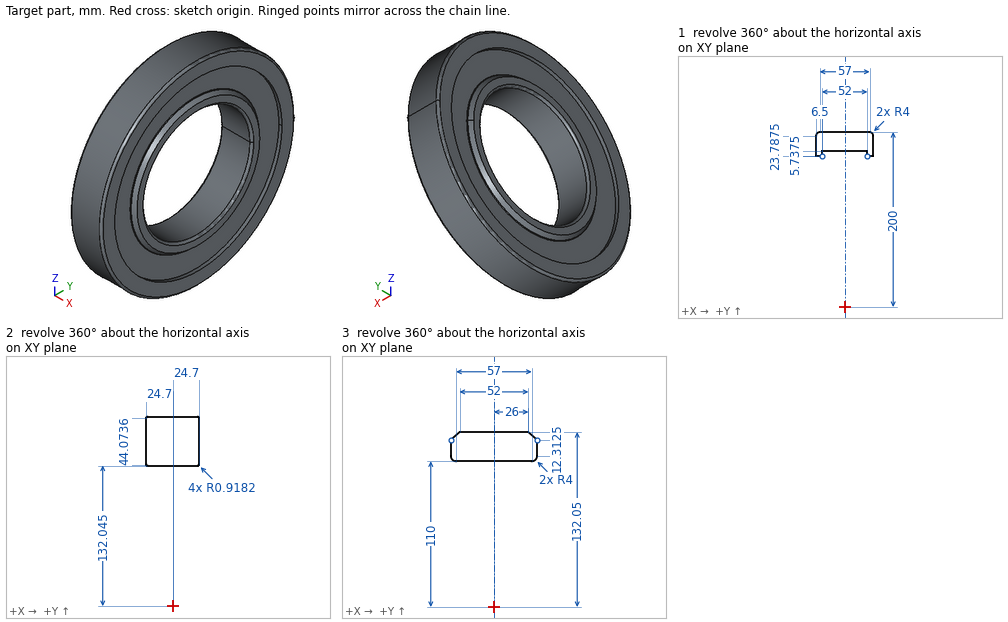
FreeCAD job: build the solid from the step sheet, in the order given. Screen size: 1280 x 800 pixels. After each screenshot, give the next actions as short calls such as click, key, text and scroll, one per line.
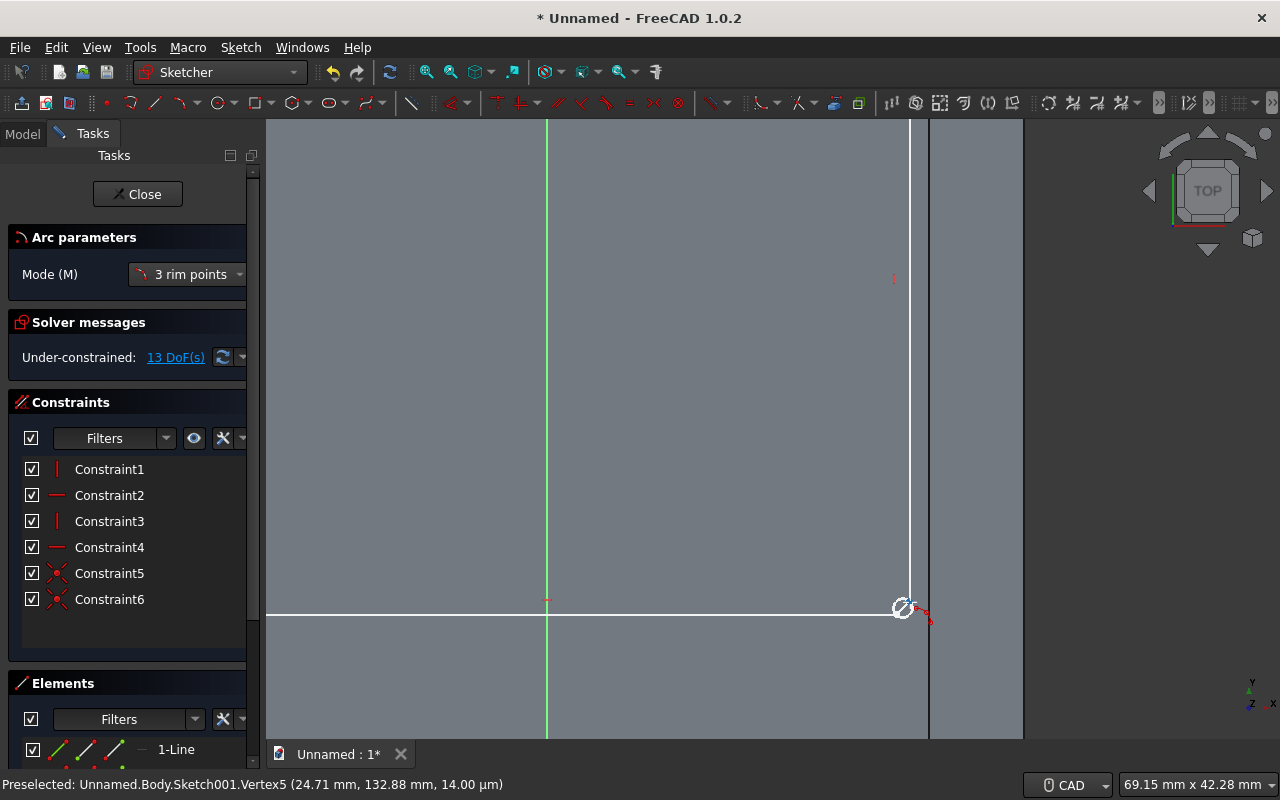
scroll(906, 610, up, 7)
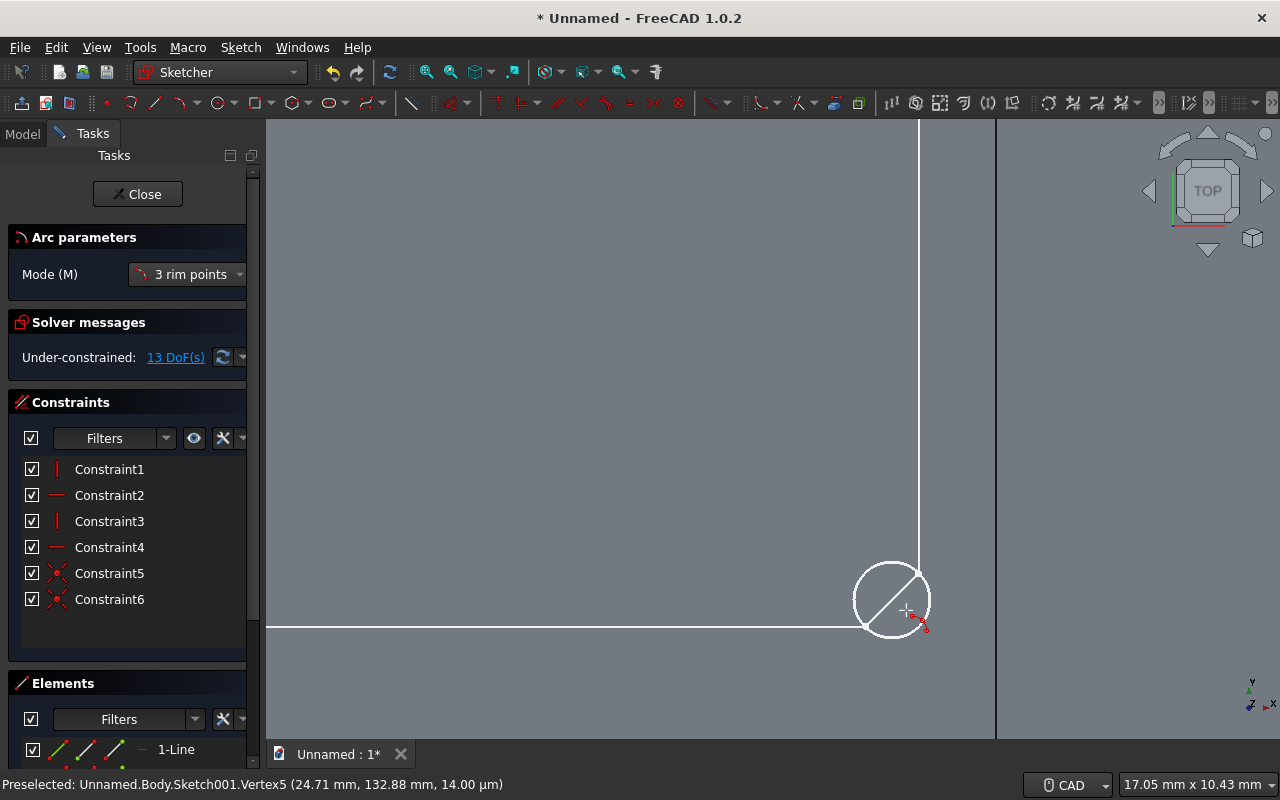
click(902, 607)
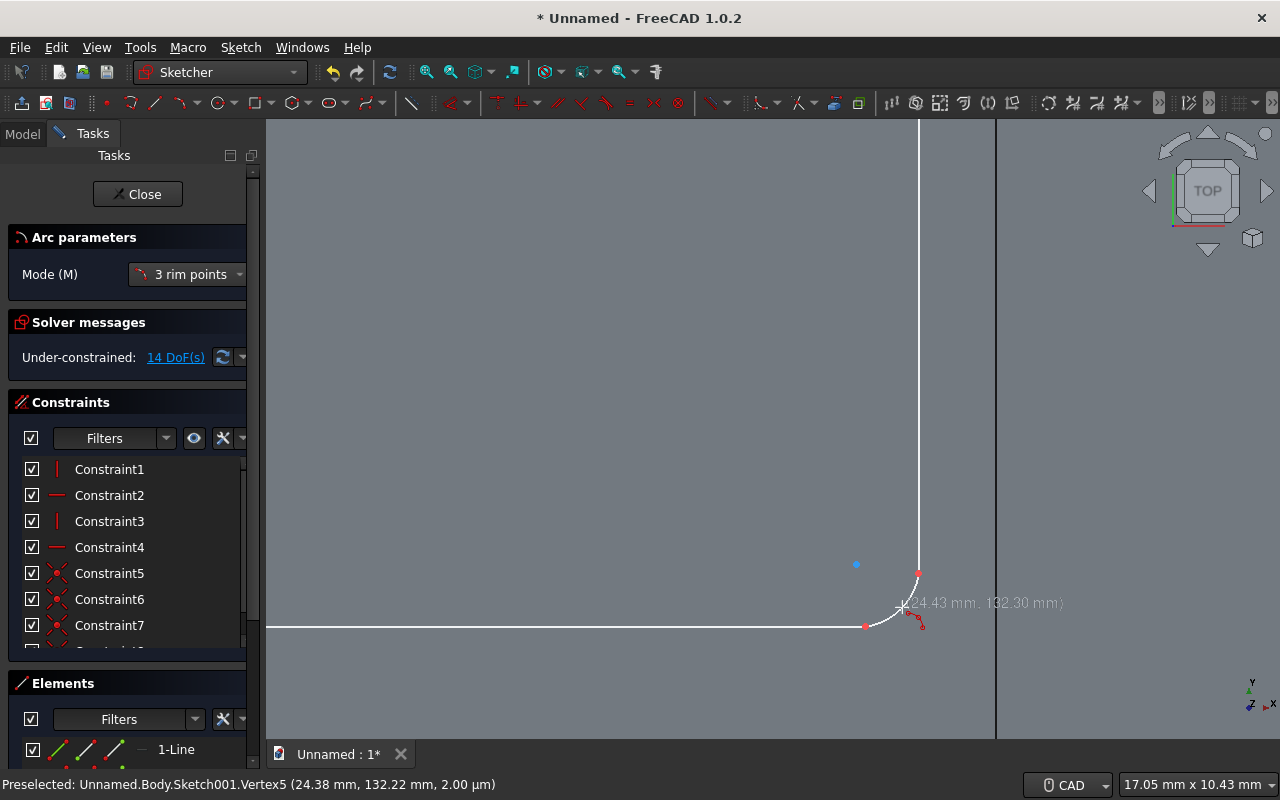
scroll(901, 612, down, 10)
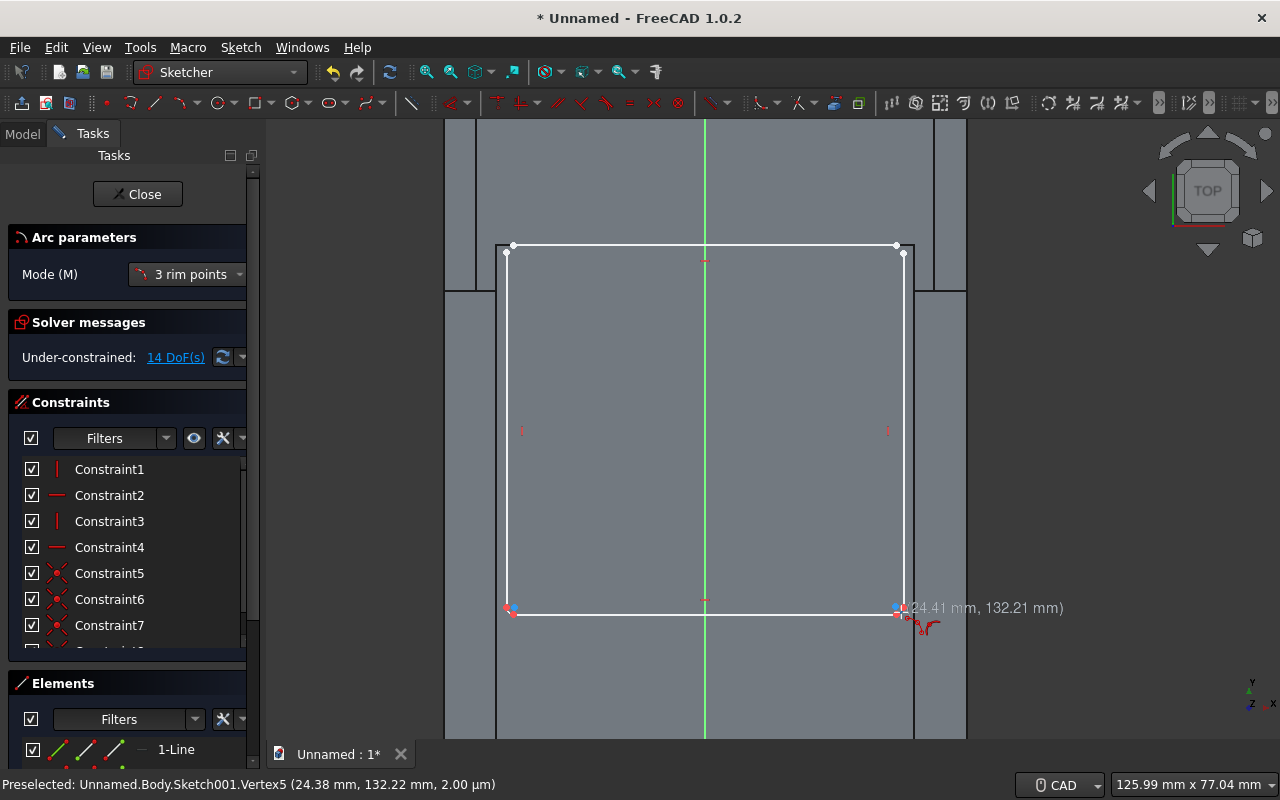
scroll(904, 252, up, 3)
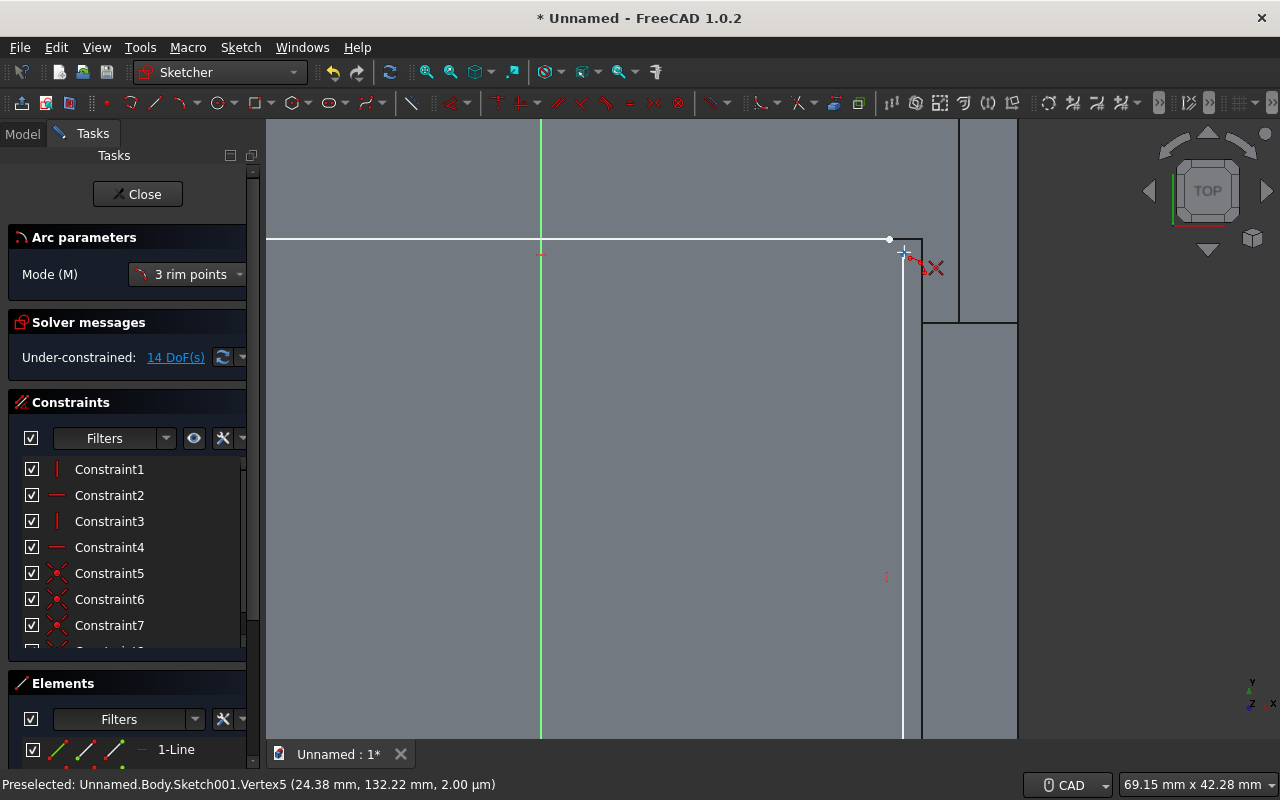
click(903, 254)
click(890, 239)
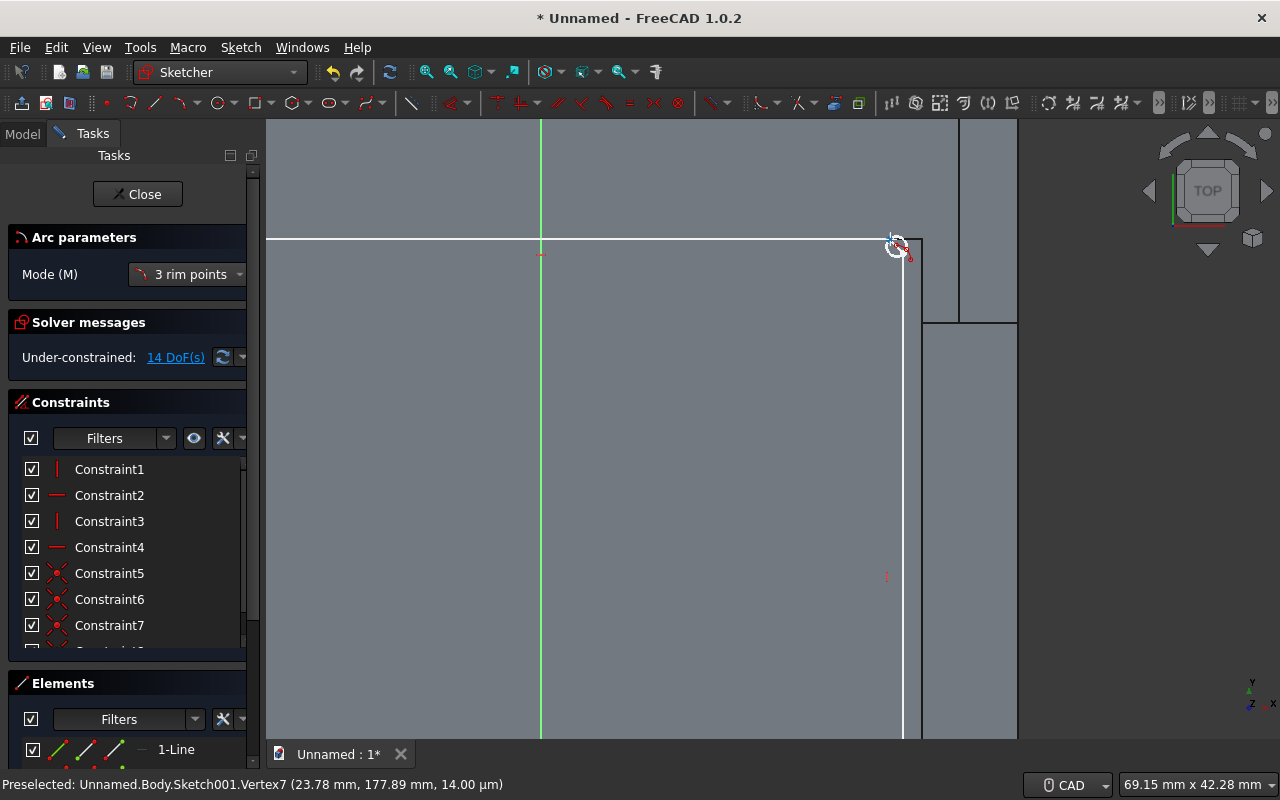
scroll(899, 242, up, 7)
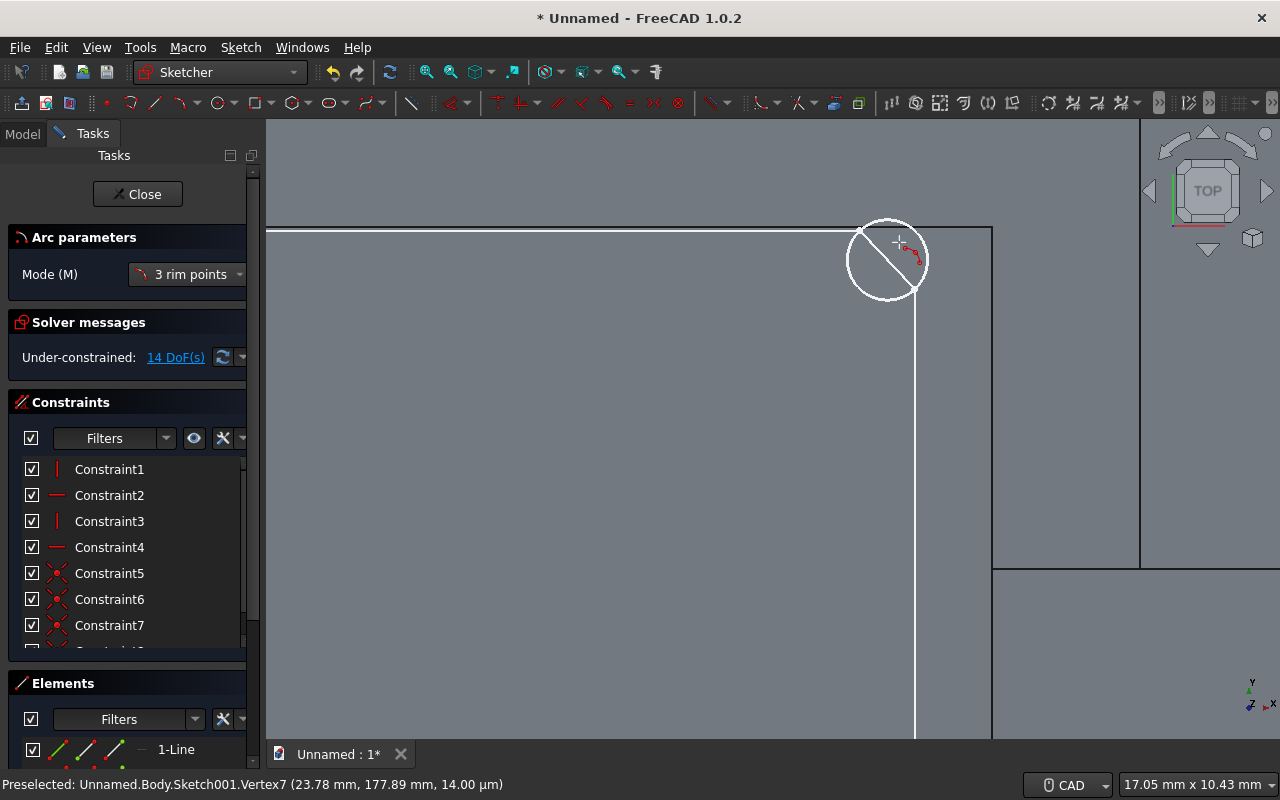
click(898, 243)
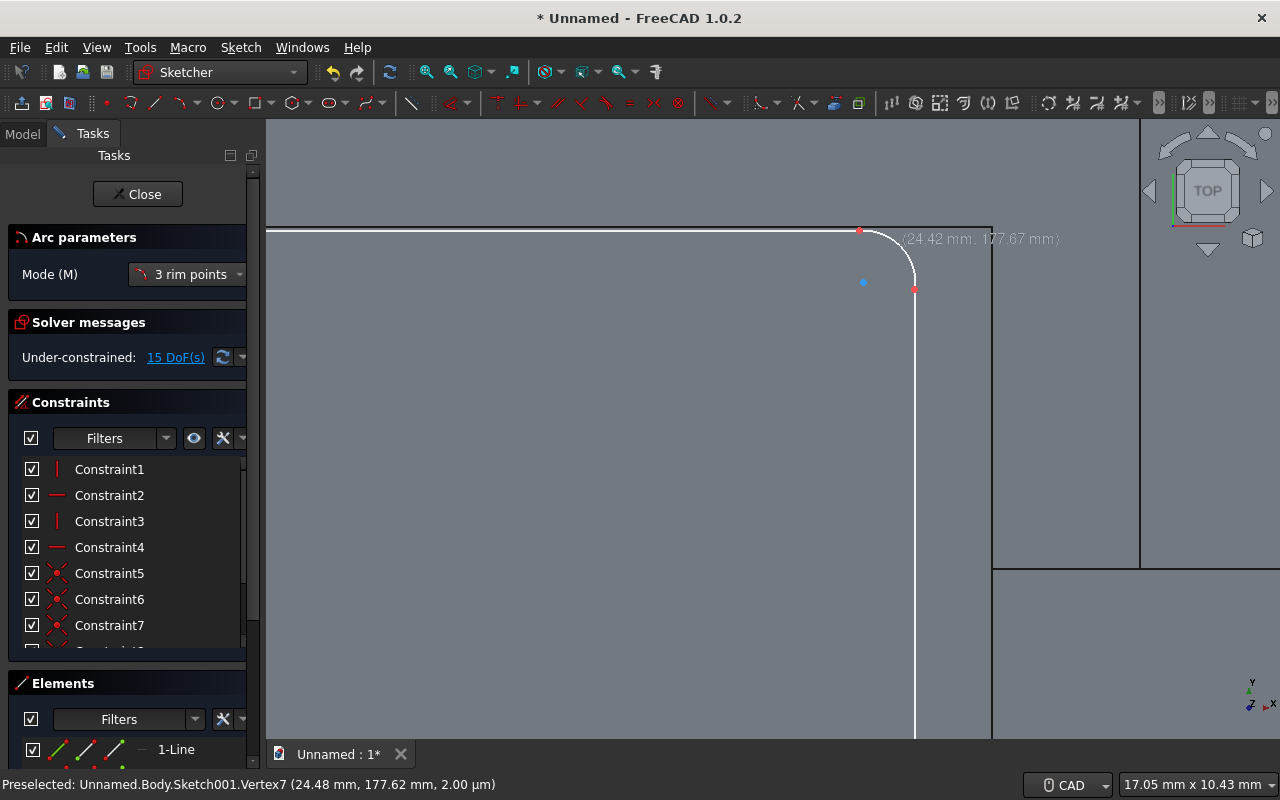
scroll(902, 247, down, 10)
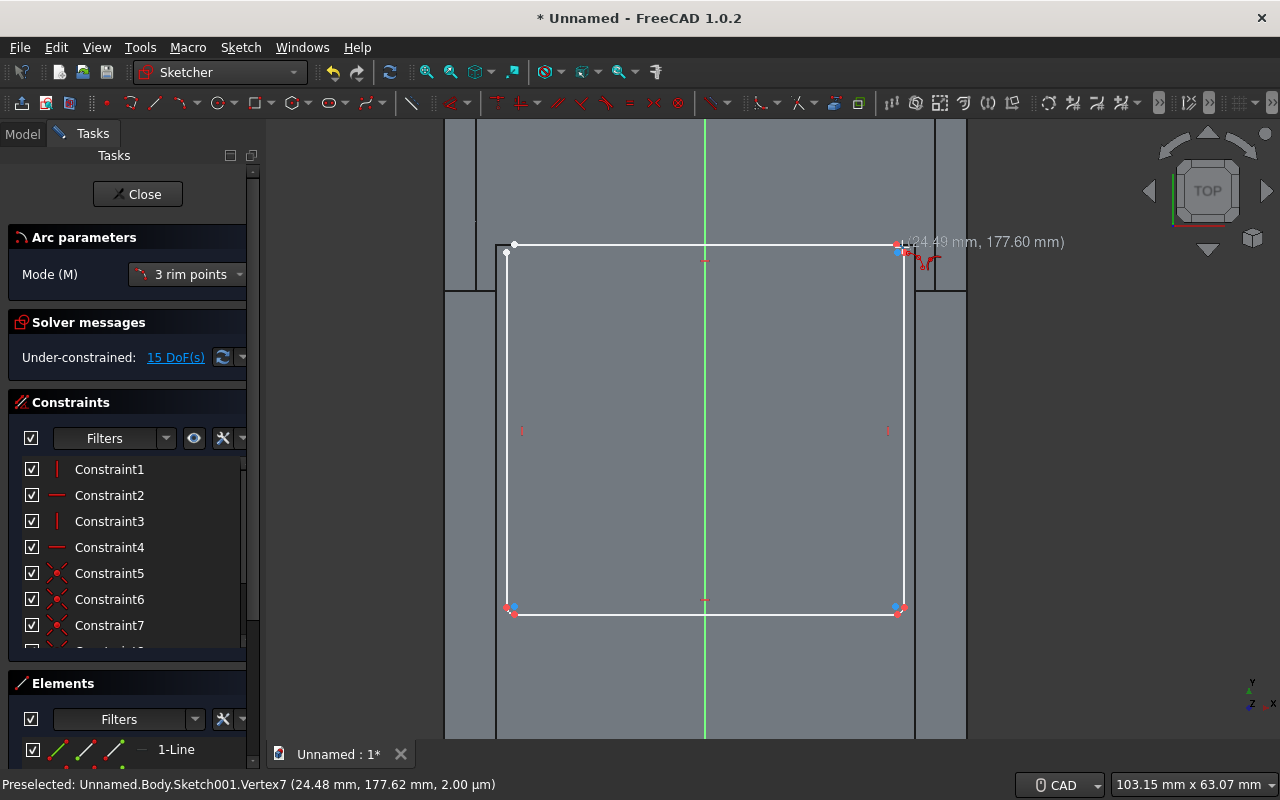
scroll(514, 244, up, 3)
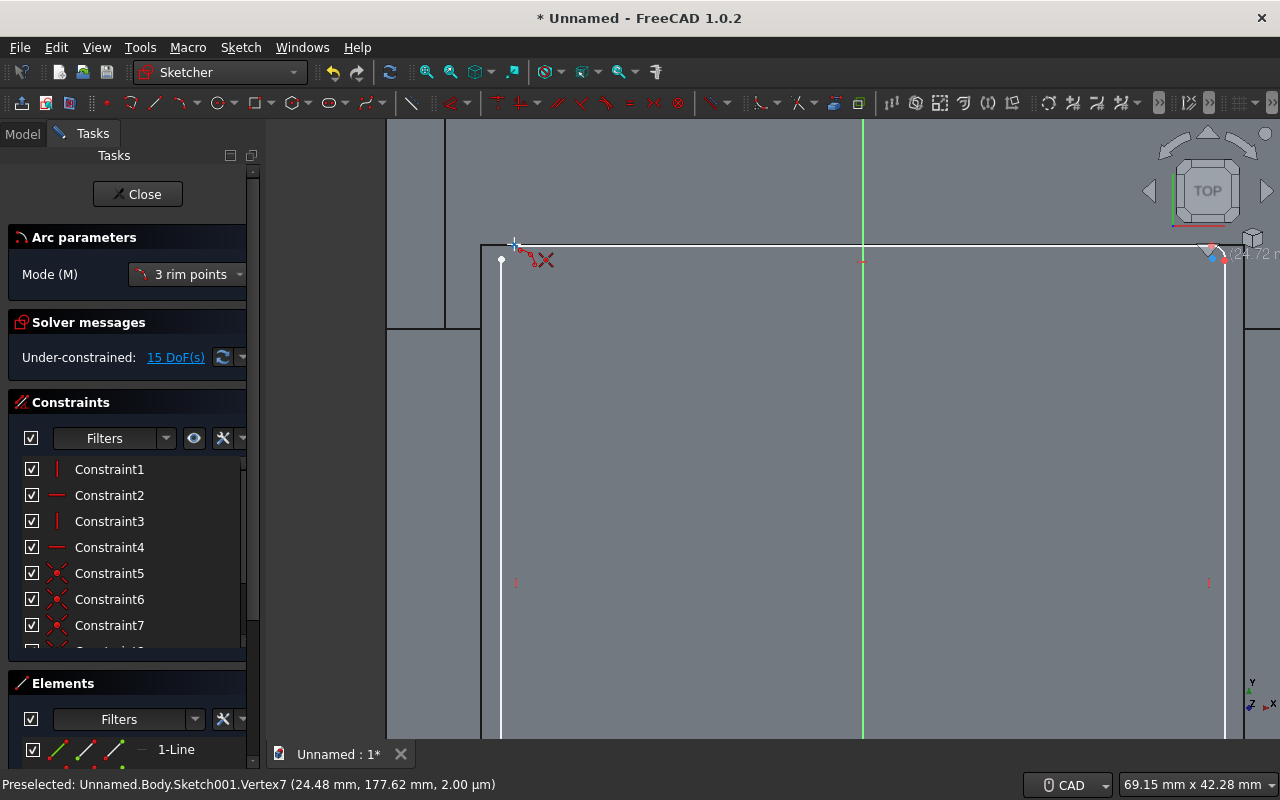
click(514, 246)
click(501, 260)